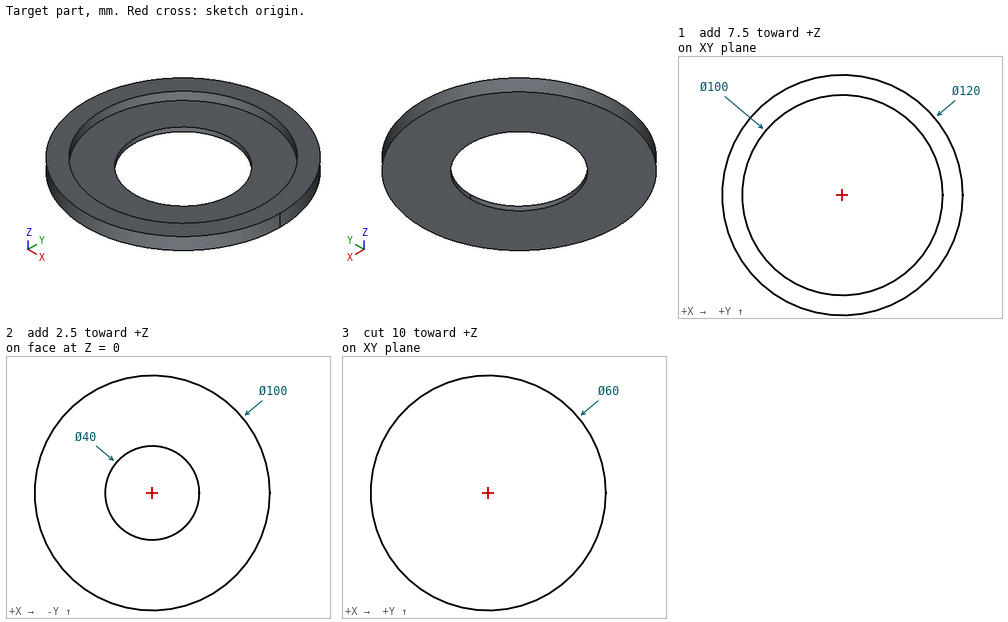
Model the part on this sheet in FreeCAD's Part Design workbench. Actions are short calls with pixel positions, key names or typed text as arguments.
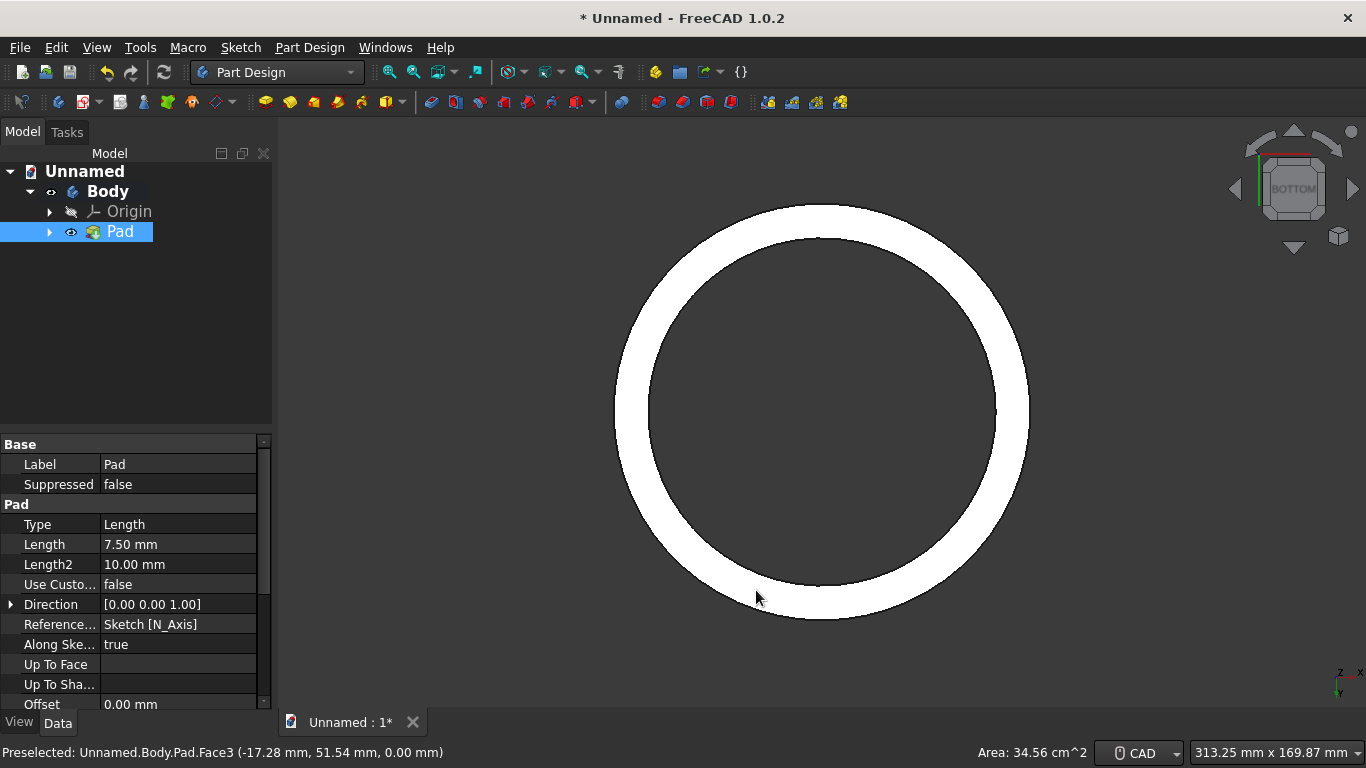
click(84, 102)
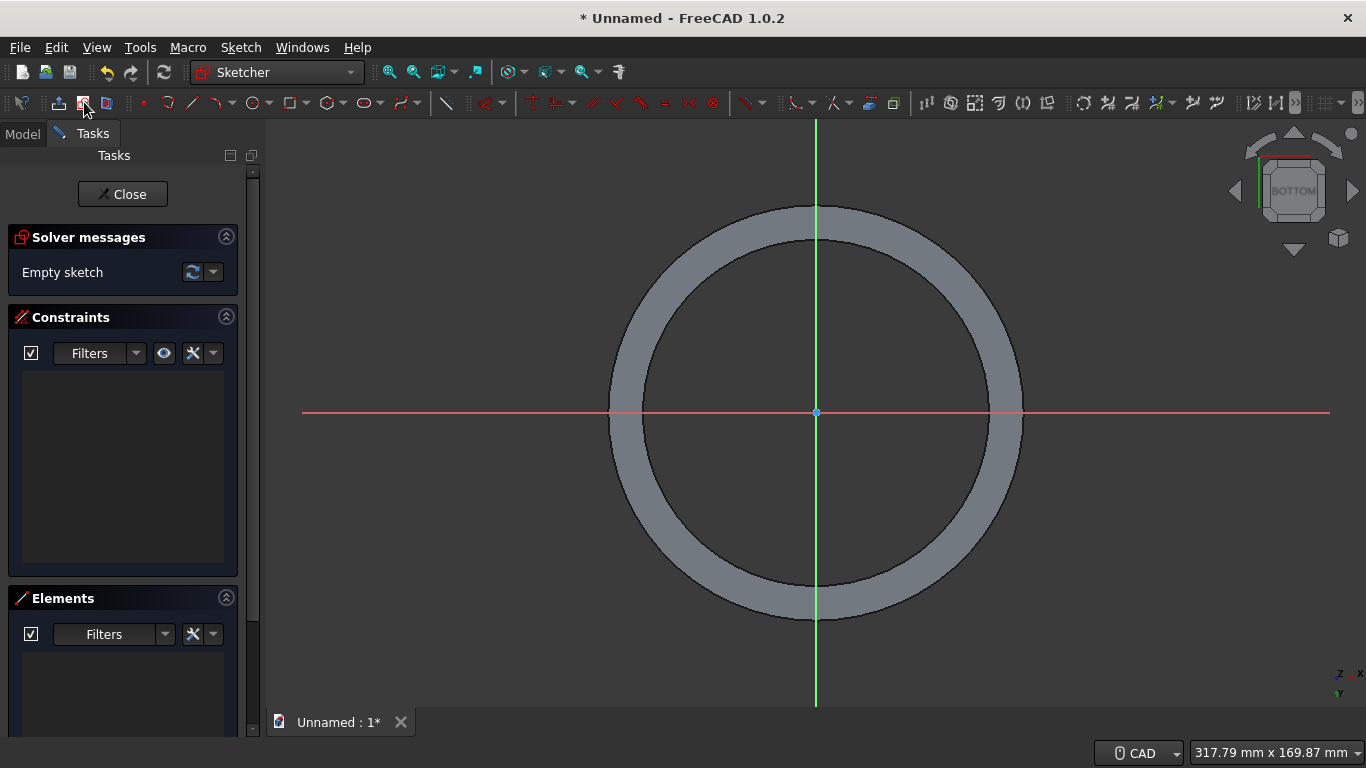
click(254, 104)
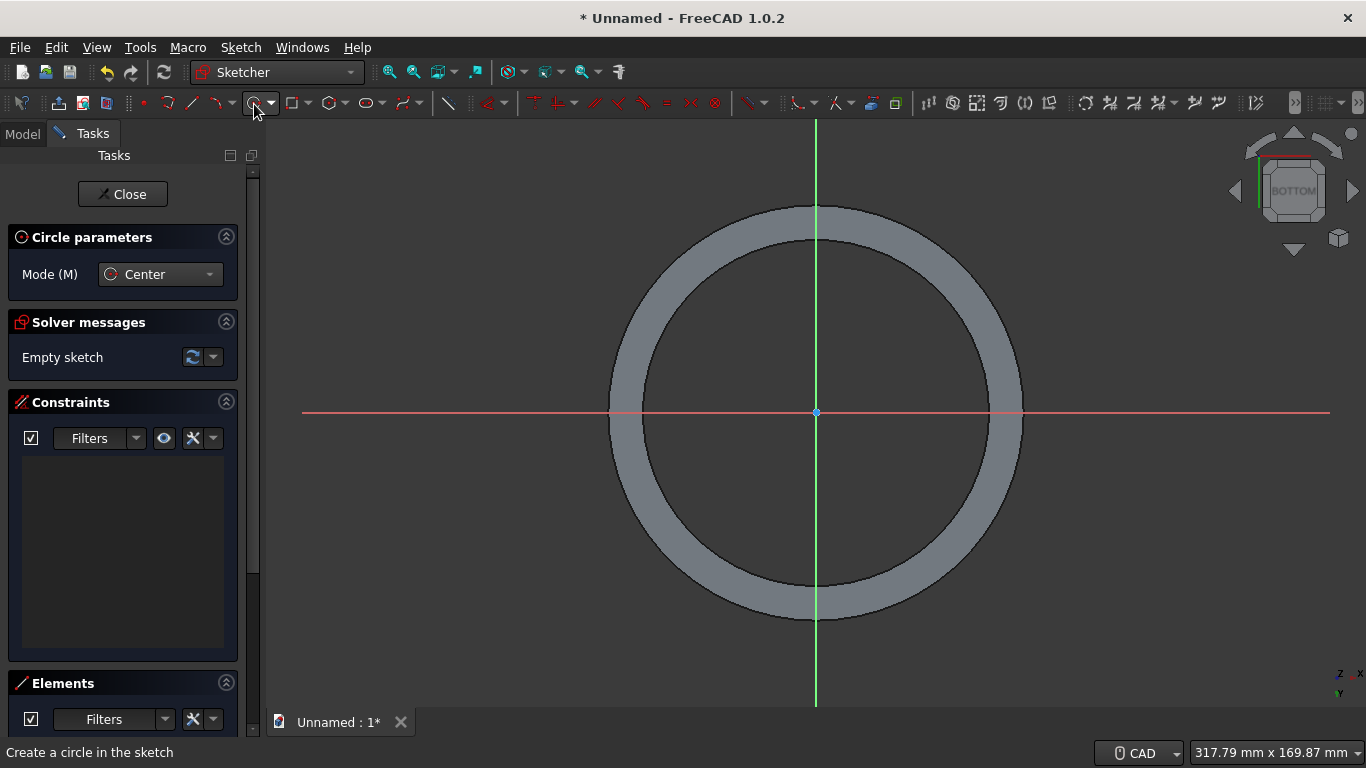
click(816, 413)
click(938, 291)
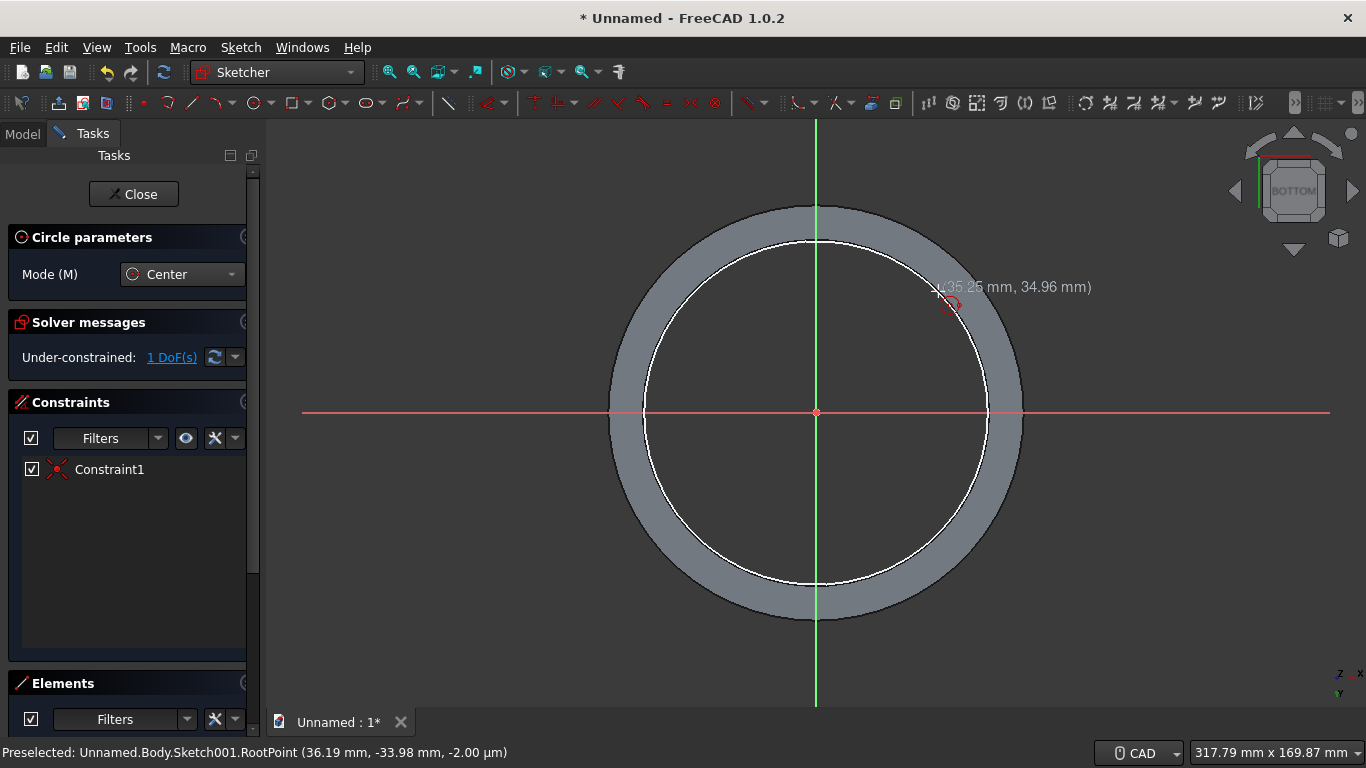
click(816, 413)
click(865, 364)
key(Escape)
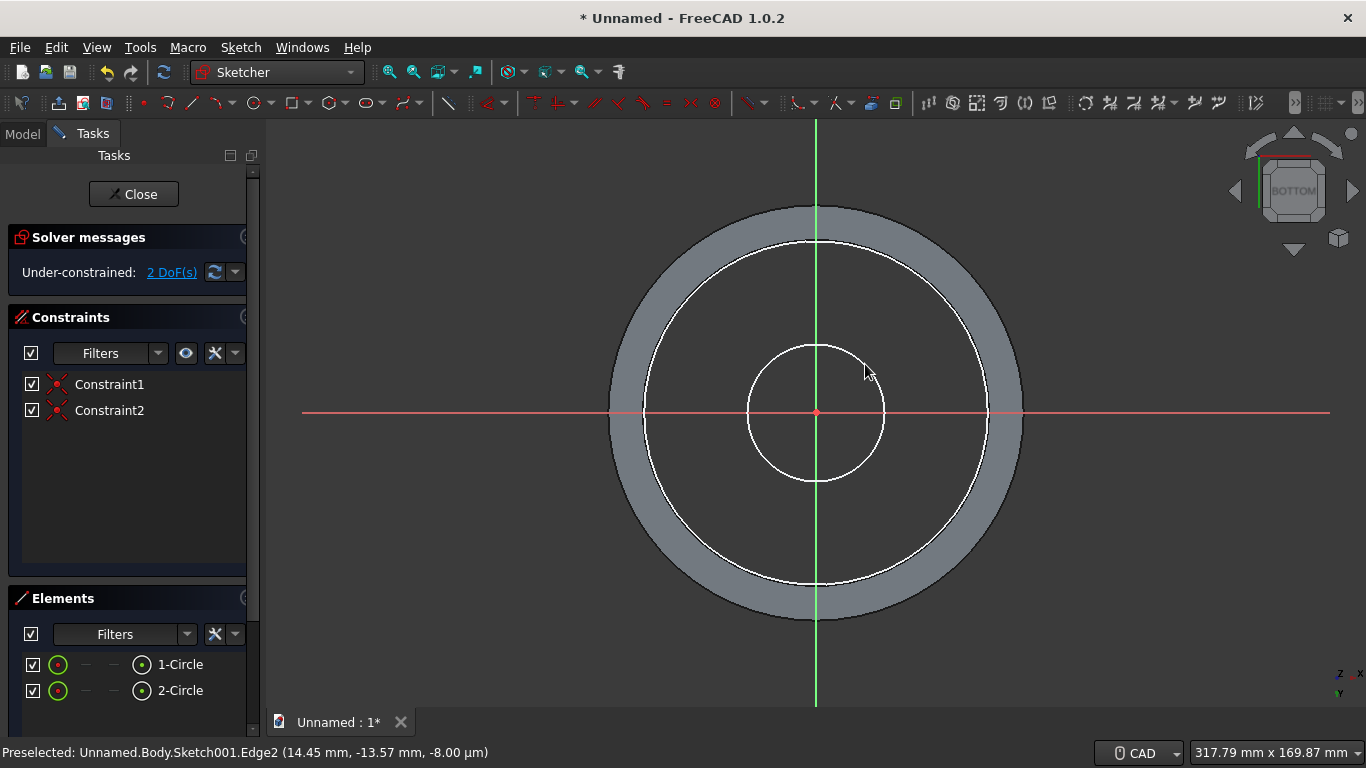
click(488, 104)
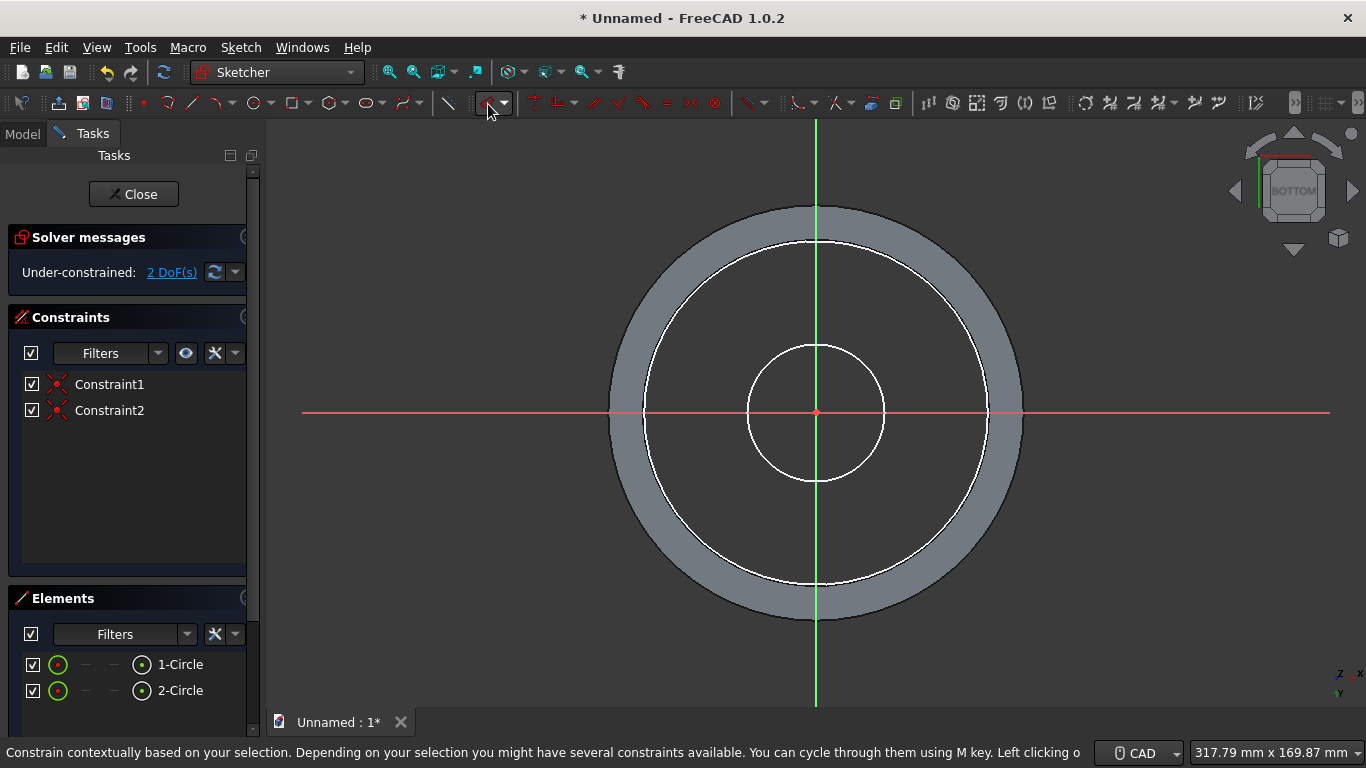
click(937, 291)
click(960, 268)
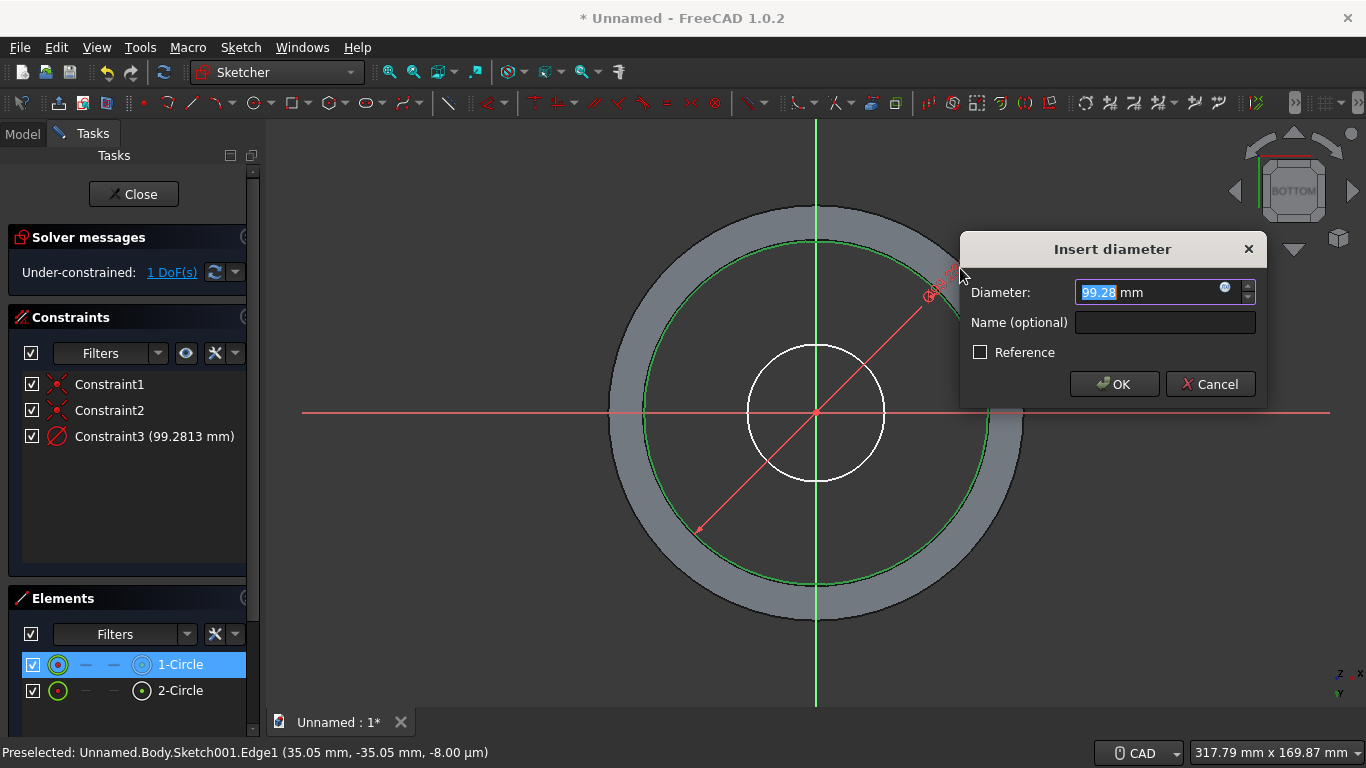
text(100)
key(Return)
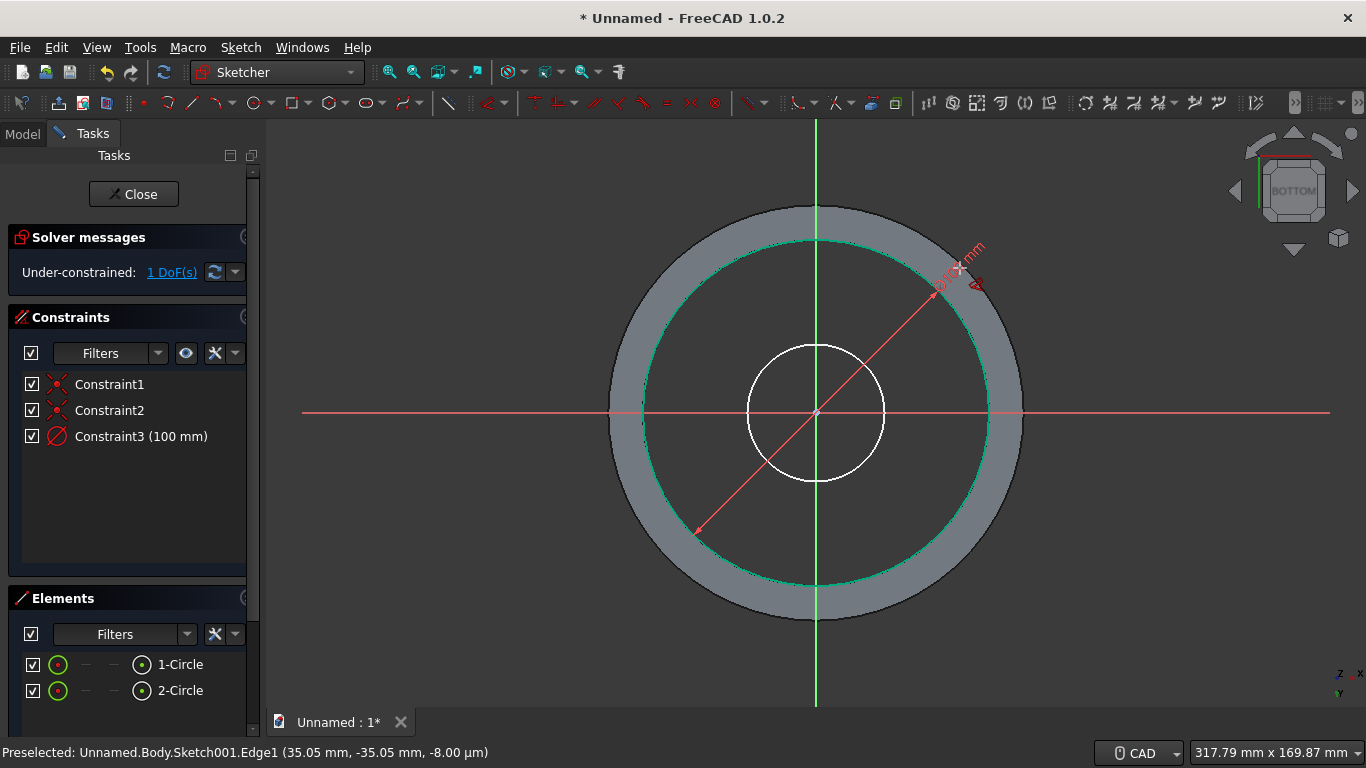
click(864, 364)
click(886, 341)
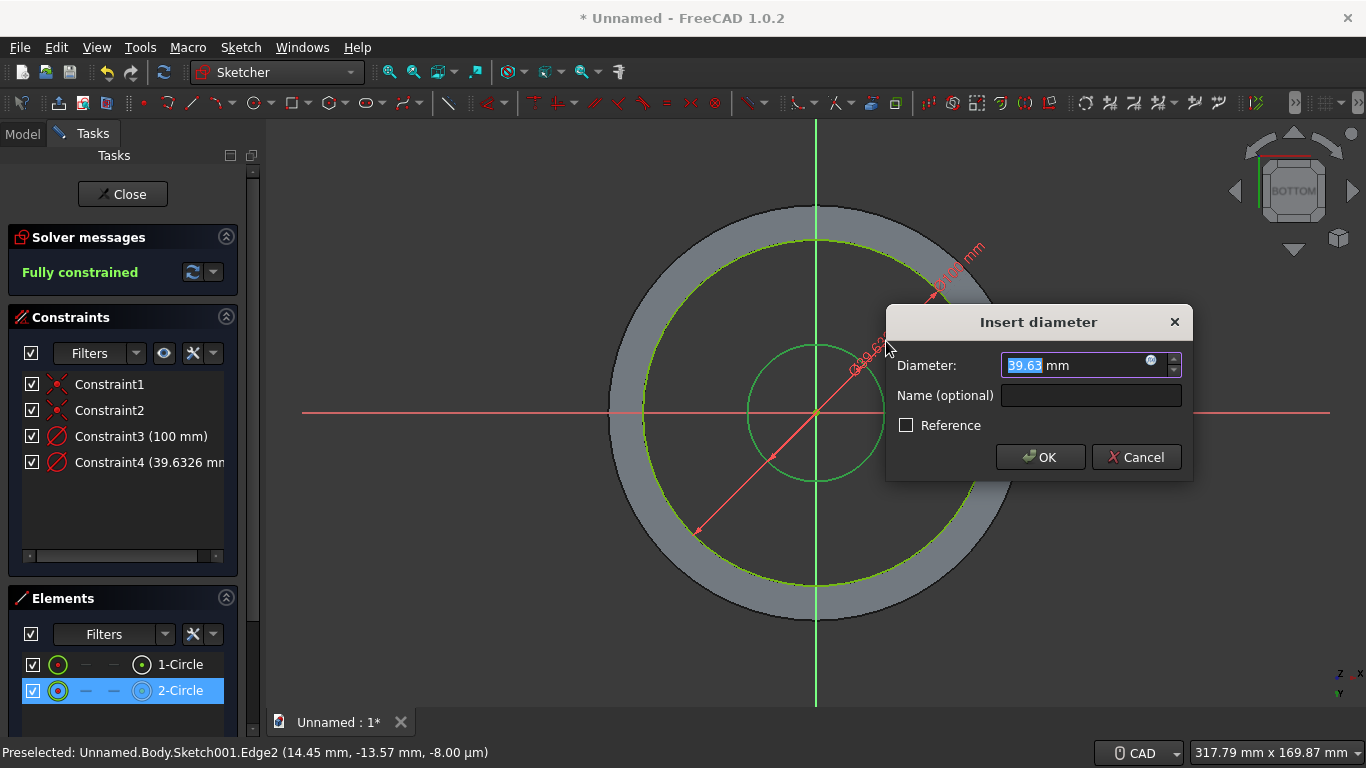
text(40)
key(Return)
key(Escape)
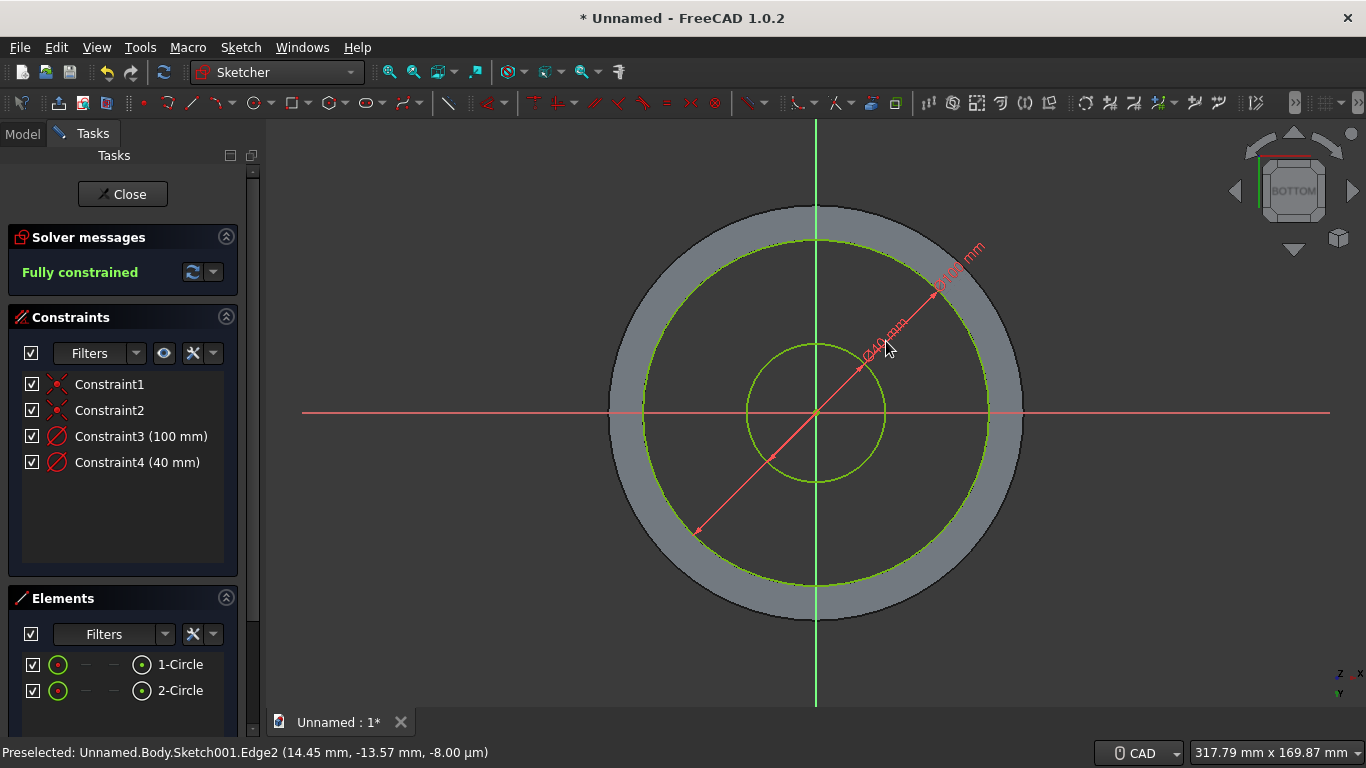
click(123, 194)